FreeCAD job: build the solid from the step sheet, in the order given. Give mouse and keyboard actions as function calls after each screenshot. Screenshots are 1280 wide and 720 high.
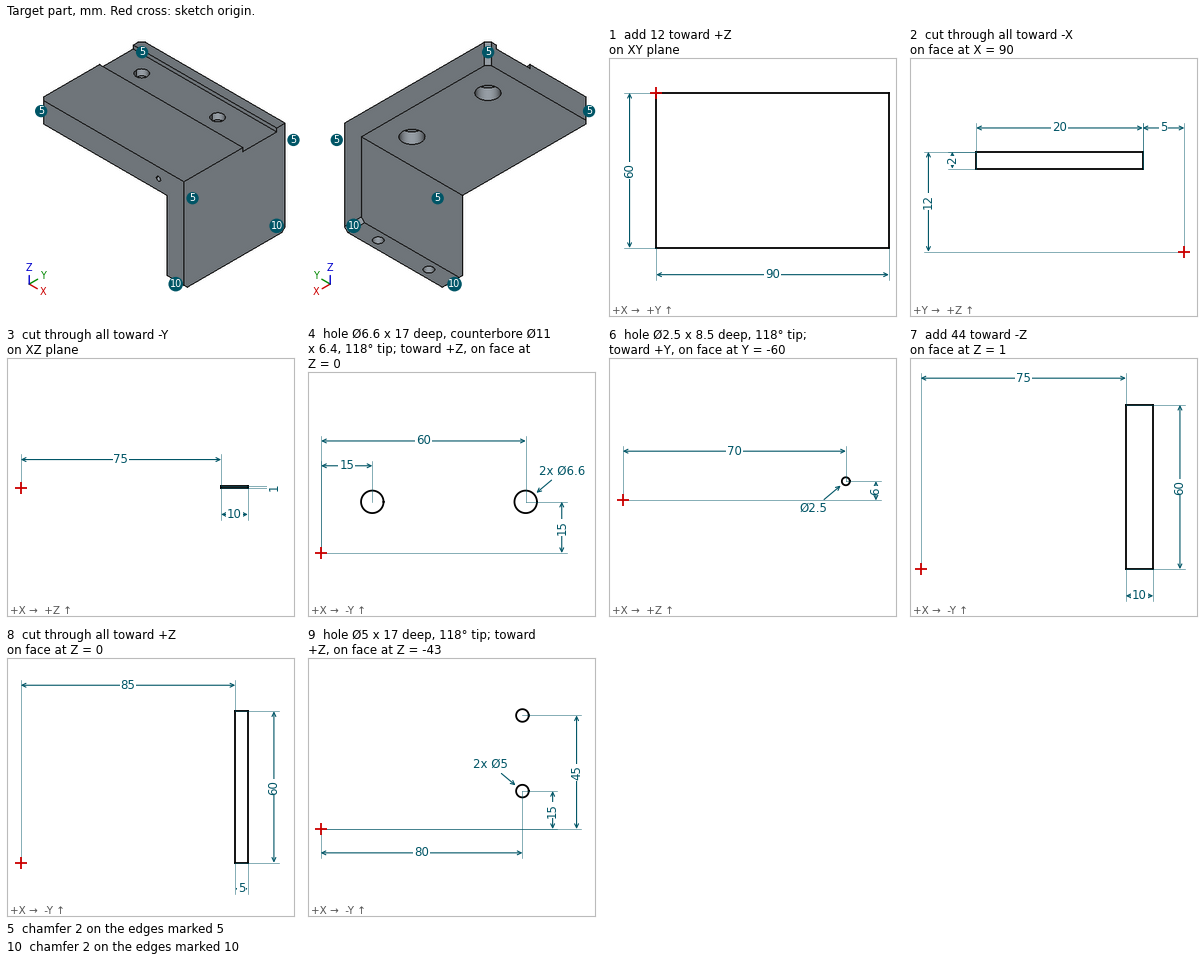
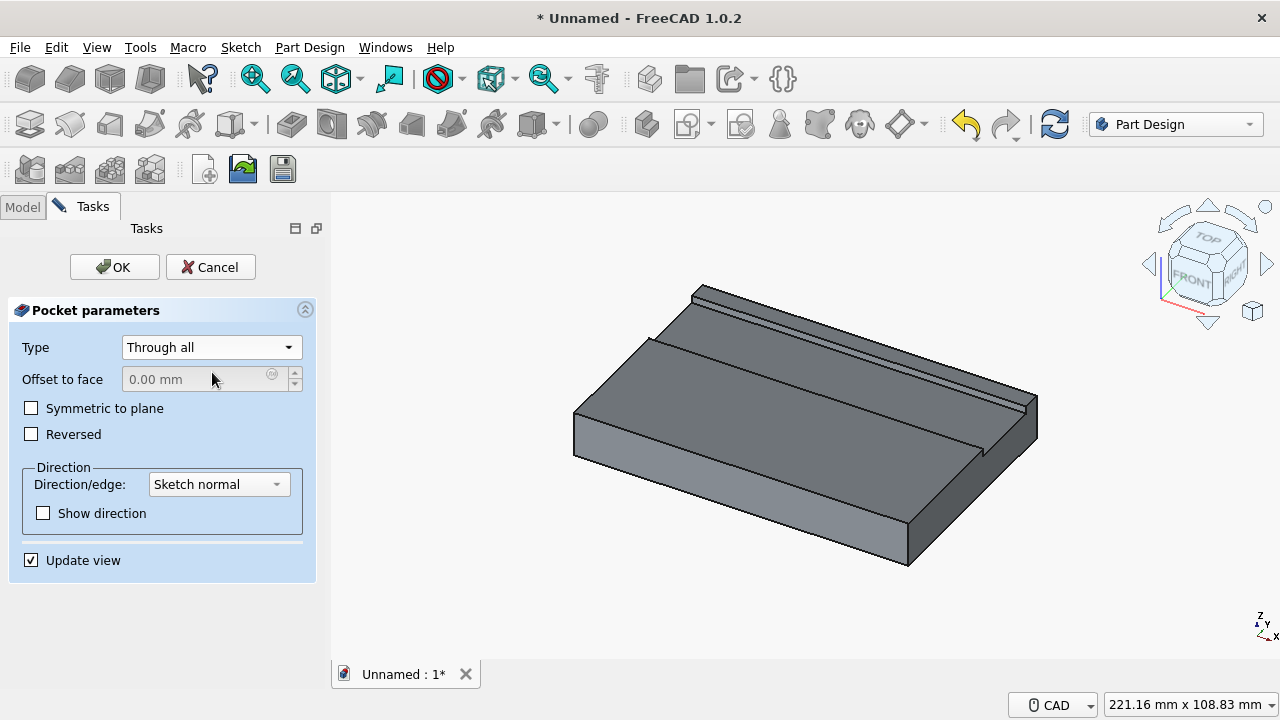
click(30, 434)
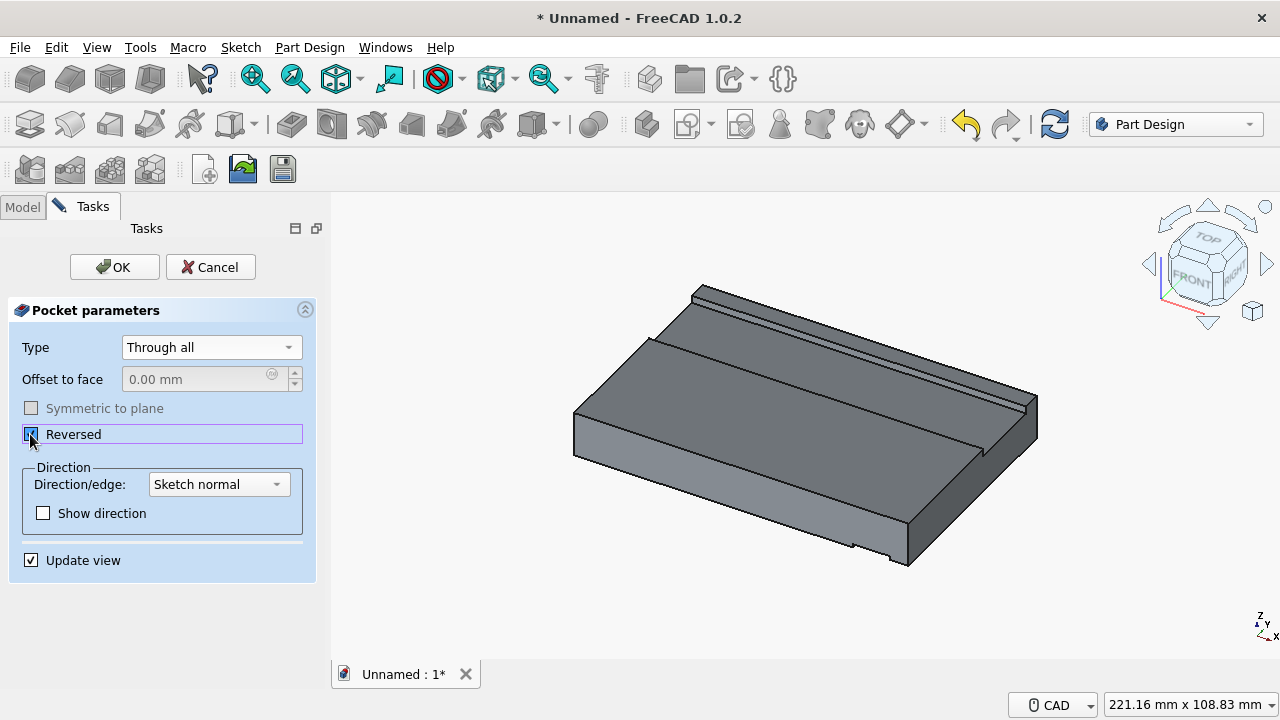
click(115, 267)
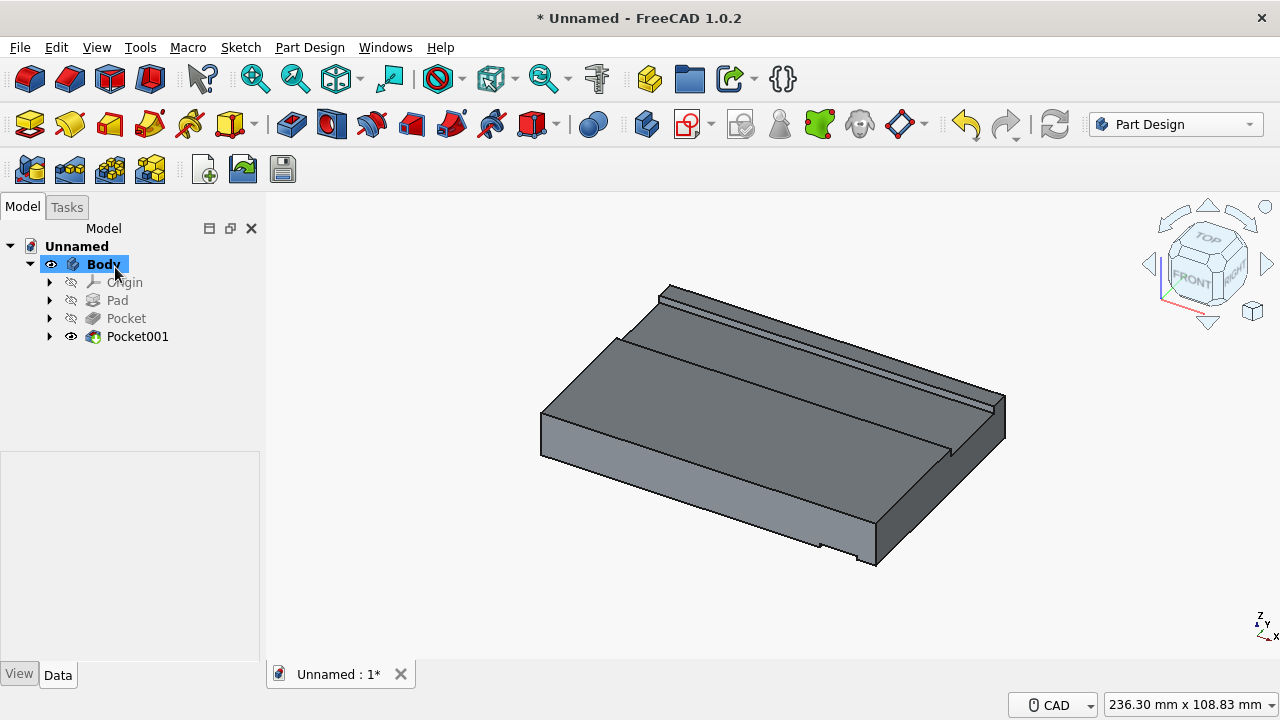
key(5)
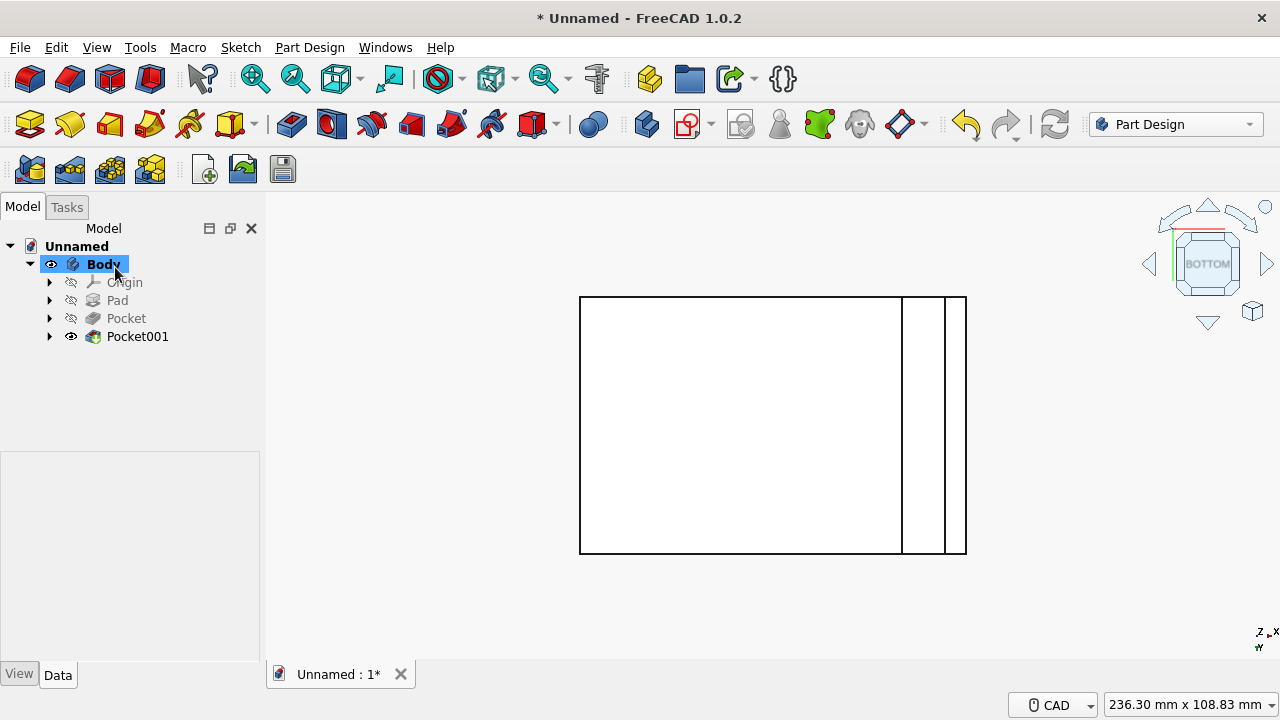
click(741, 424)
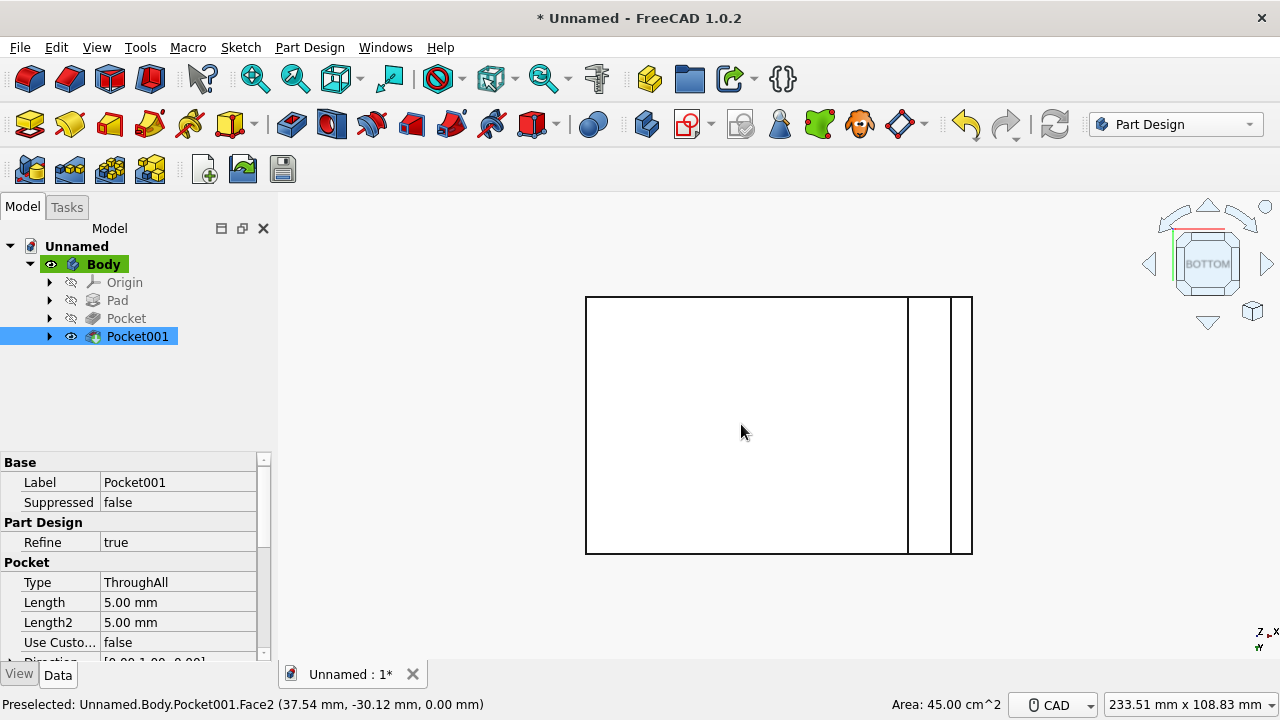
click(688, 124)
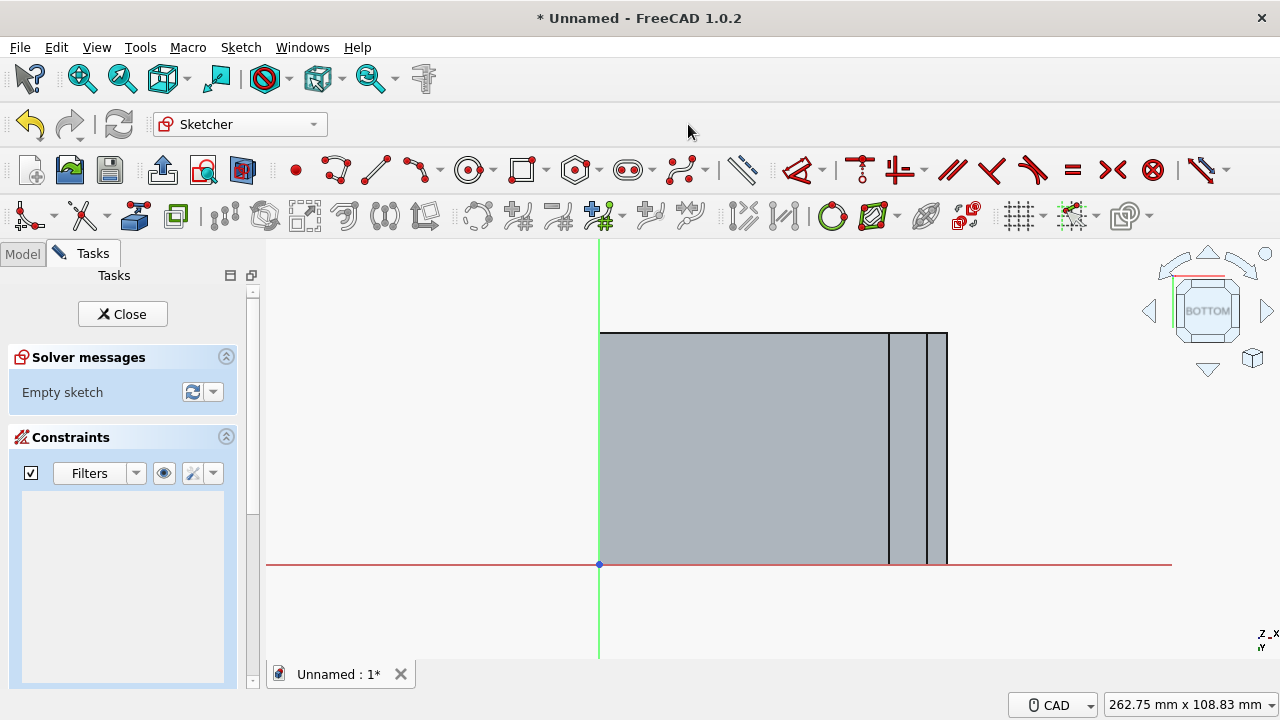
scroll(735, 595, up, 4)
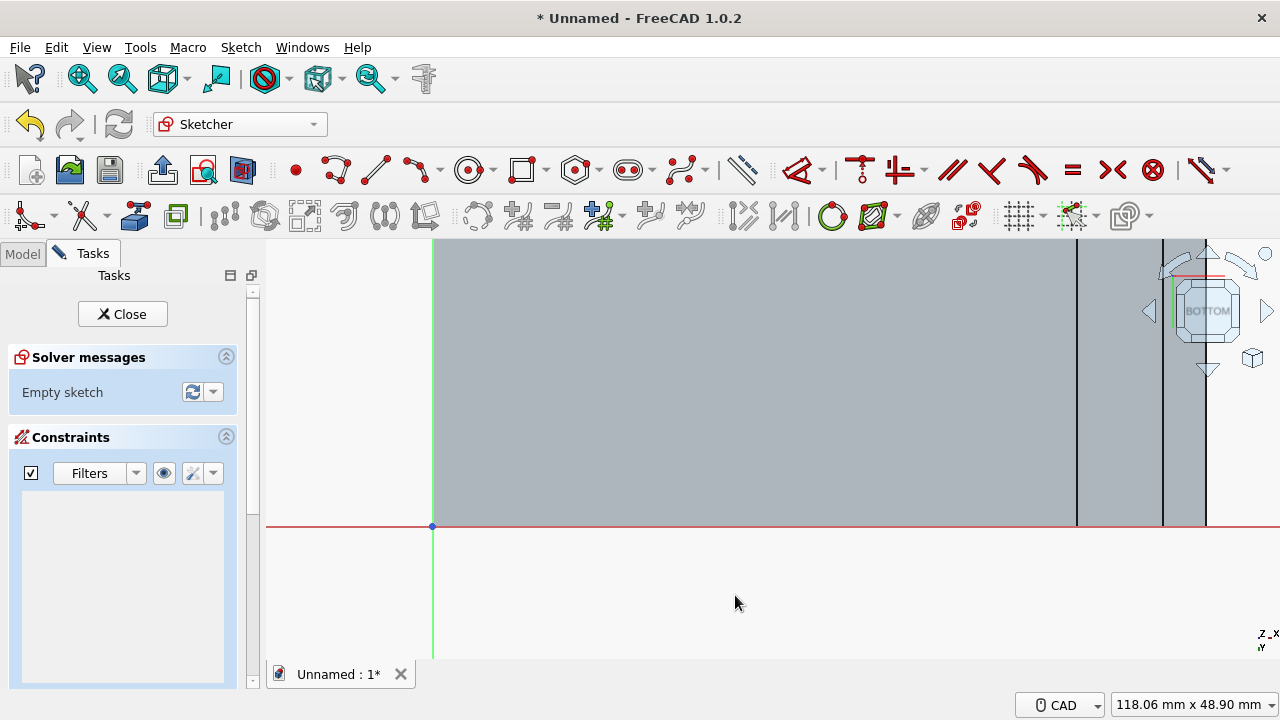
click(470, 170)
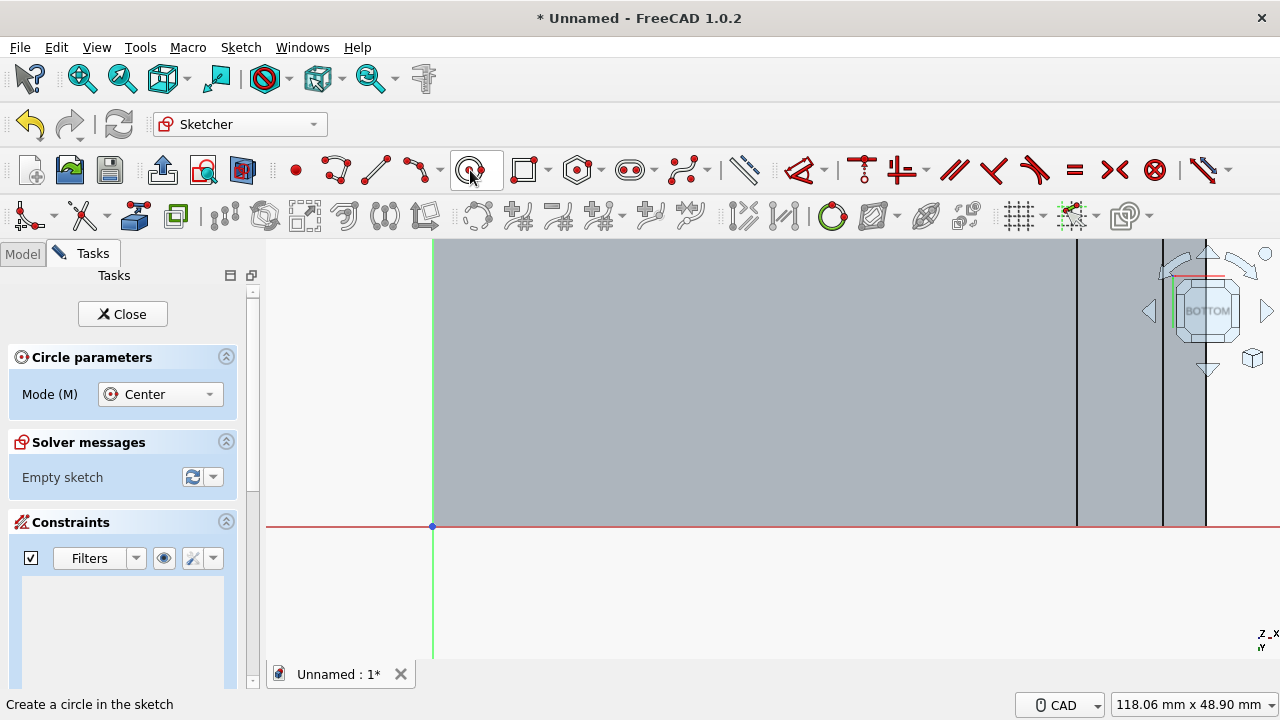
click(948, 398)
click(968, 378)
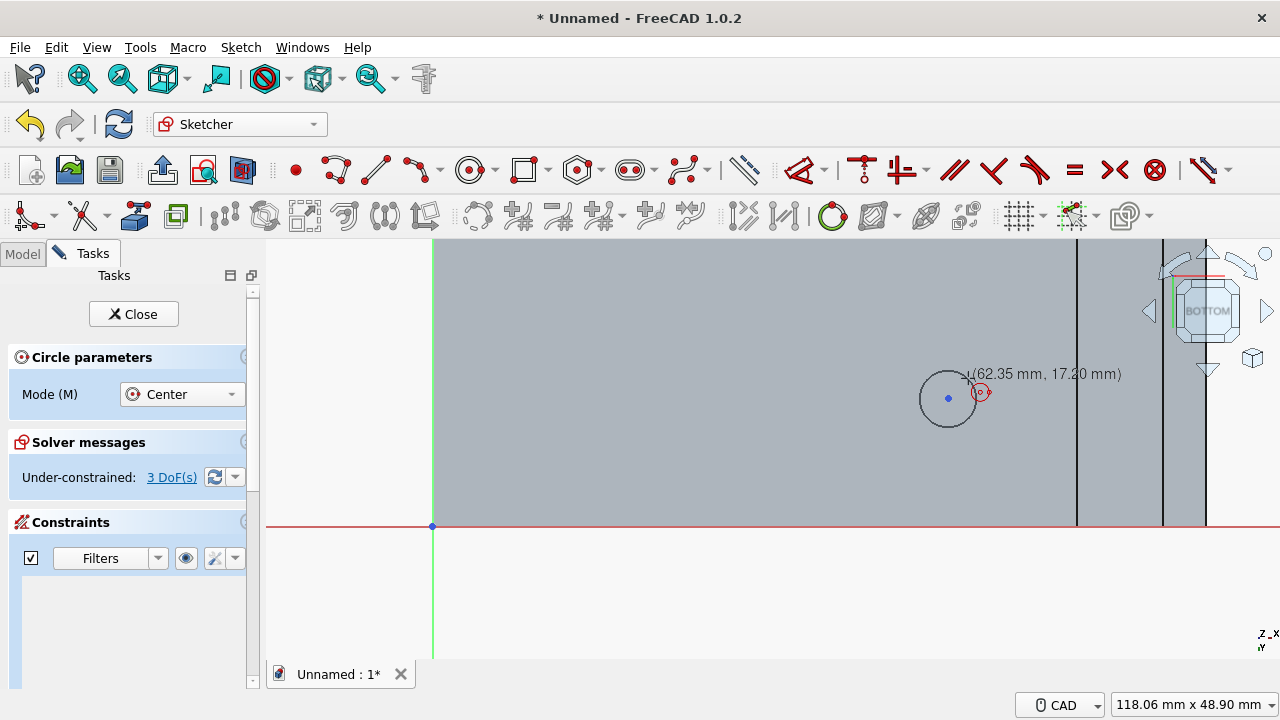
click(561, 398)
click(581, 378)
key(Escape)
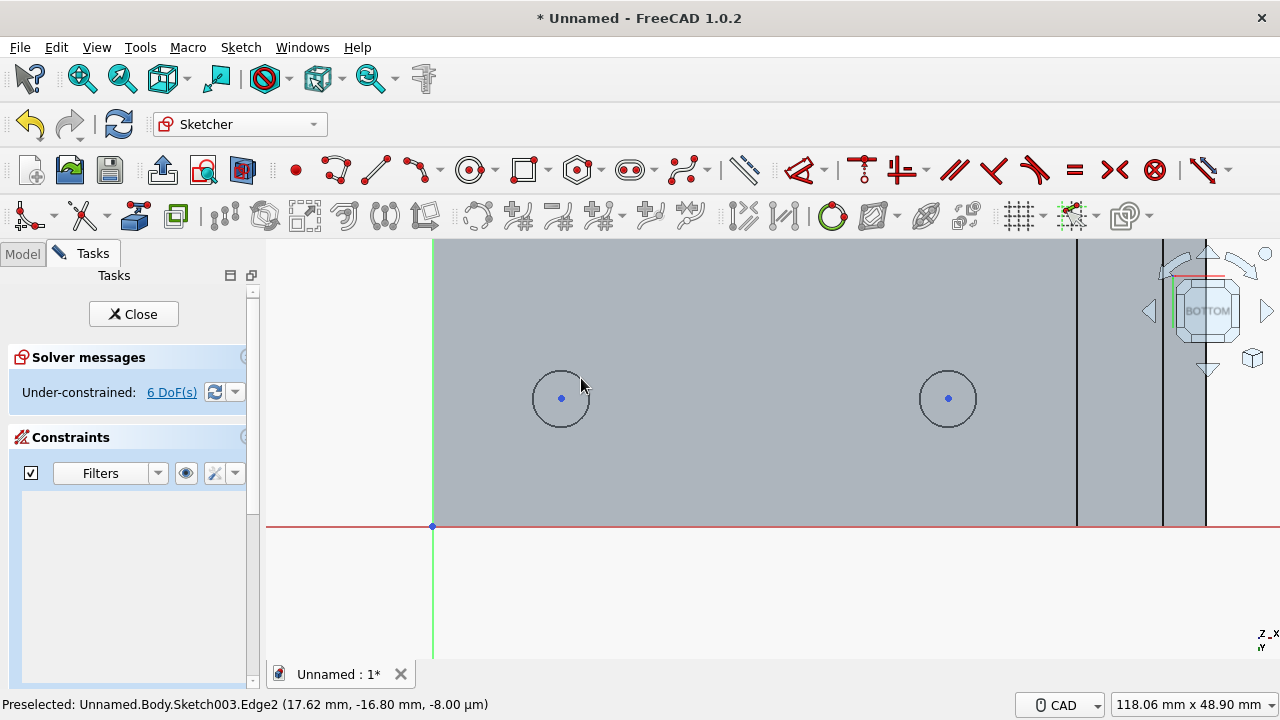
click(968, 379)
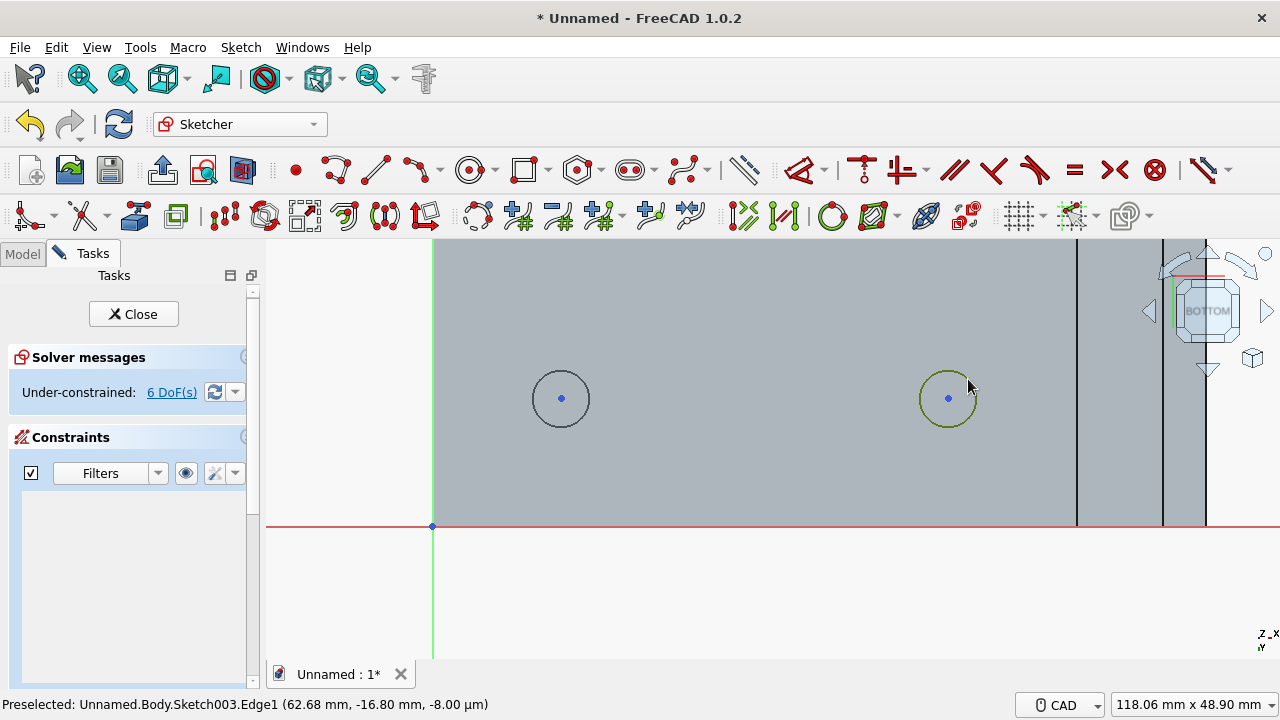
click(581, 379)